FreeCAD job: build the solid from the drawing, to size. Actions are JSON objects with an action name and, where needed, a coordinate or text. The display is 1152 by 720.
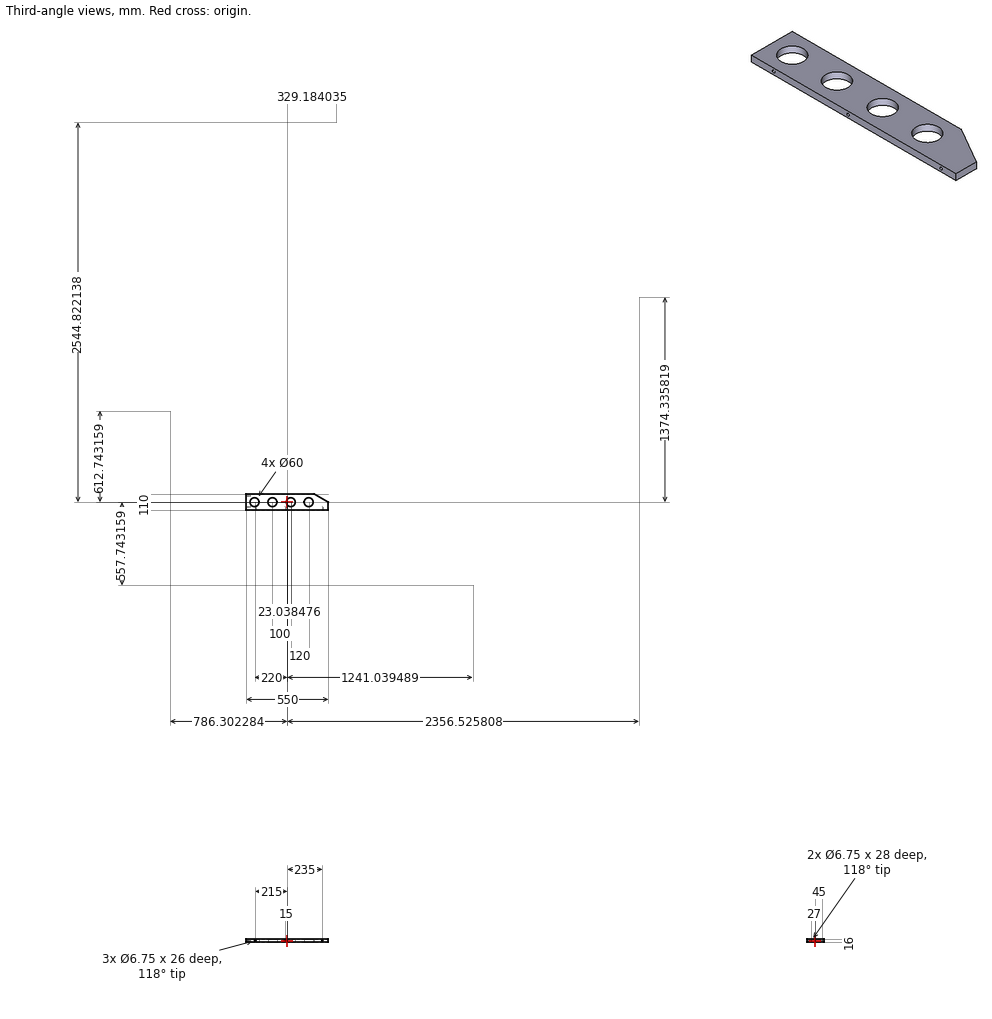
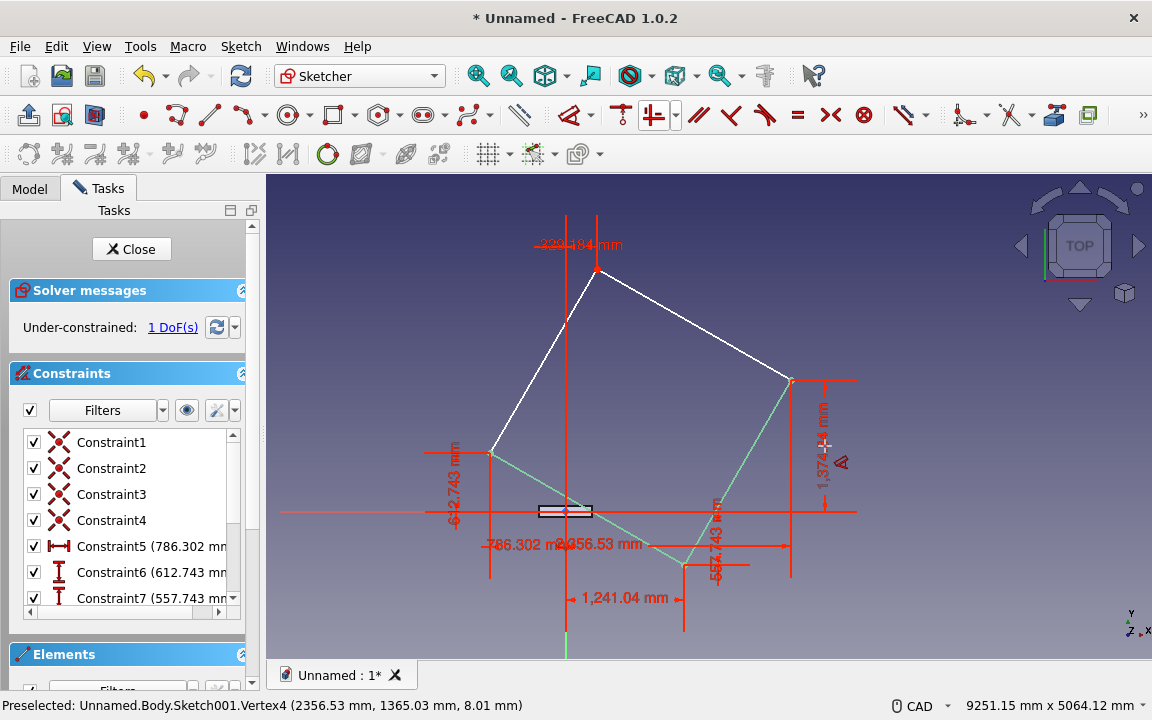
{"action": "left_click", "coordinate": [597, 269]}
{"action": "left_click", "coordinate": [532, 335]}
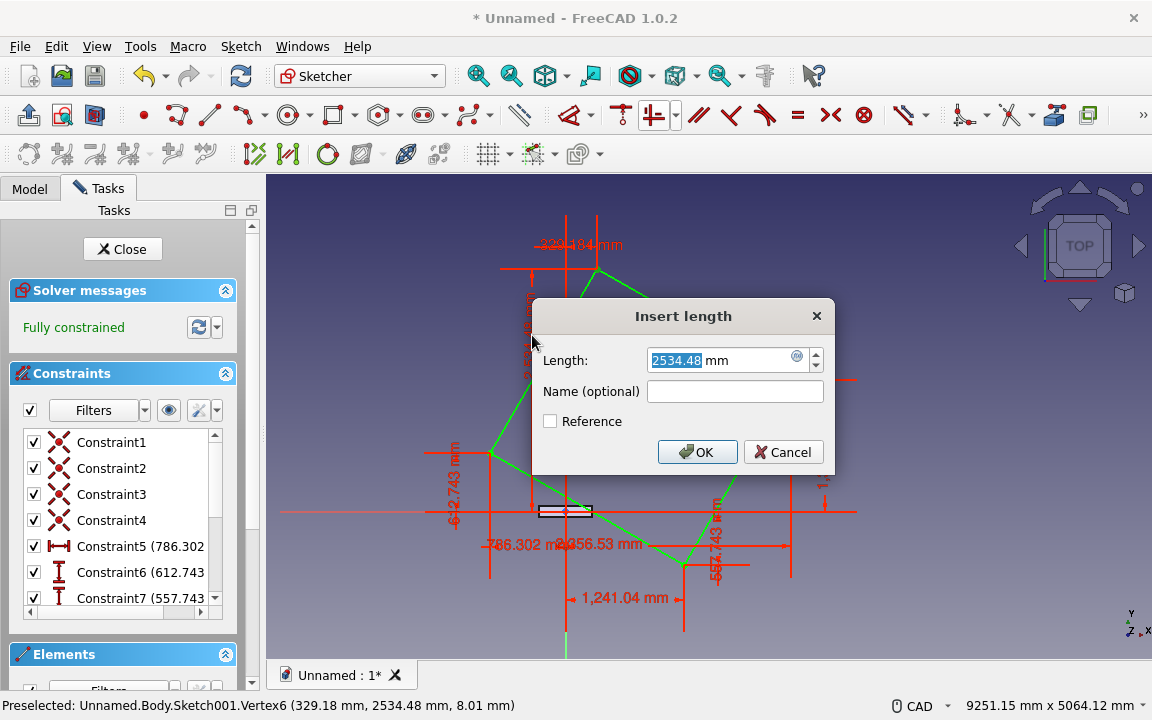
{"action": "type", "text": "2544.822138"}
{"action": "key", "text": "Return"}
{"action": "key", "text": "Escape"}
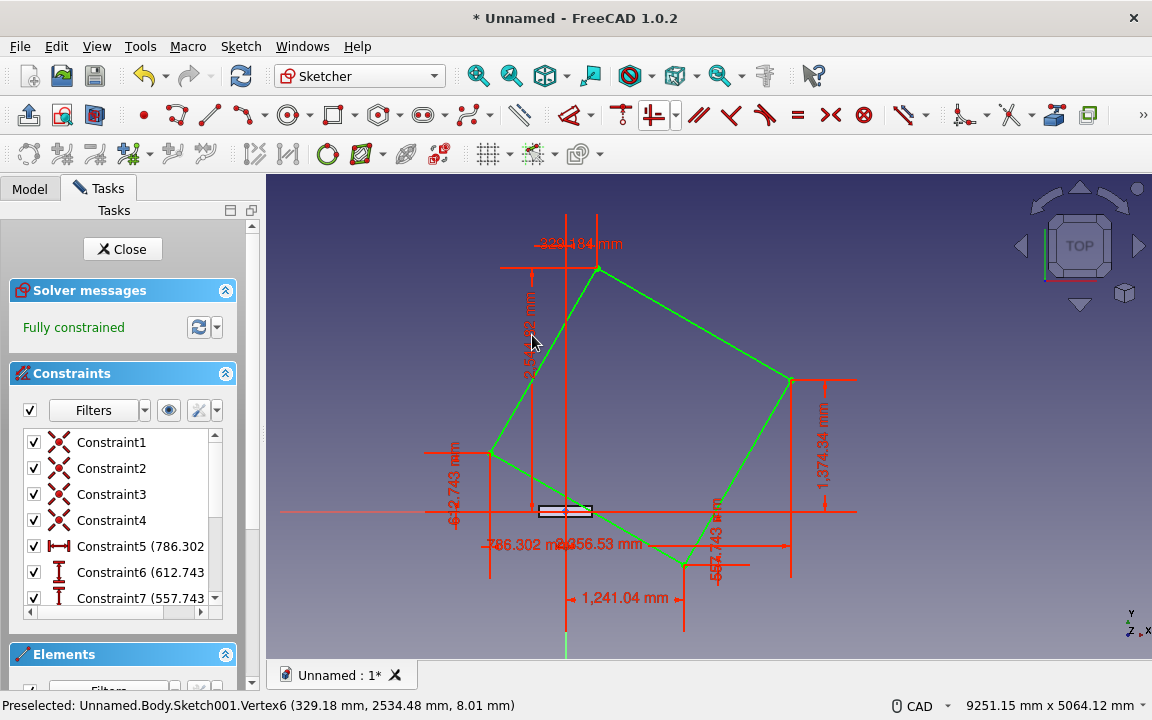
{"action": "left_click", "coordinate": [123, 249]}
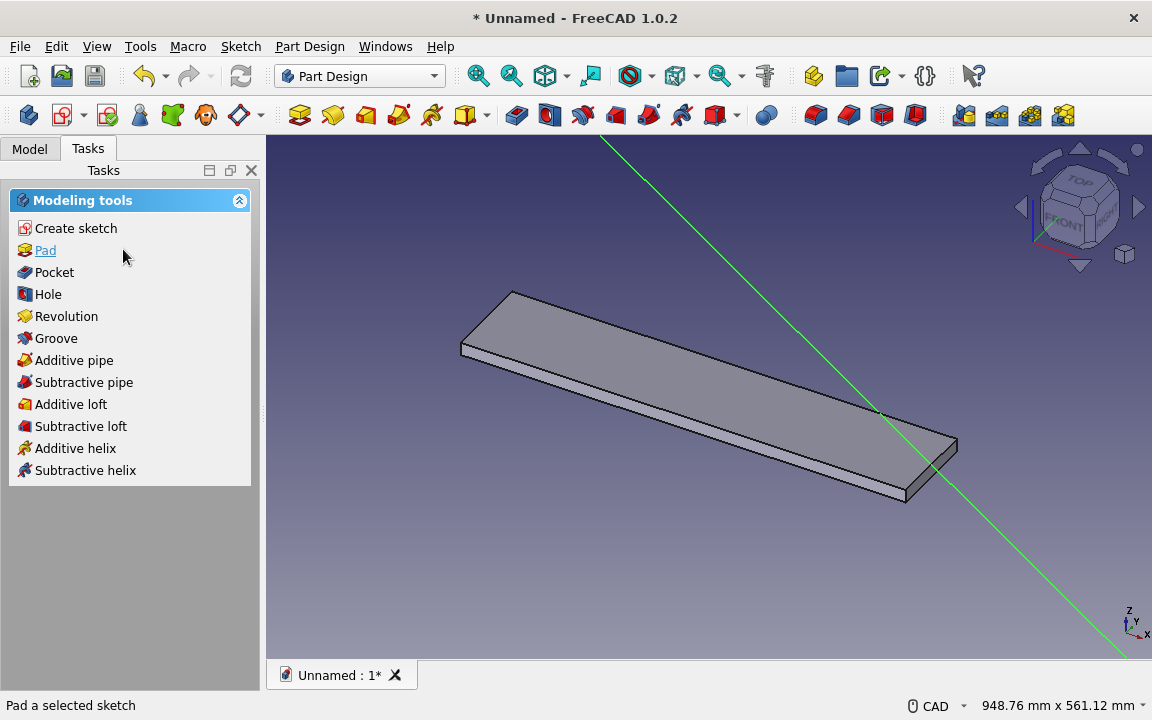
{"action": "left_click", "coordinate": [517, 116]}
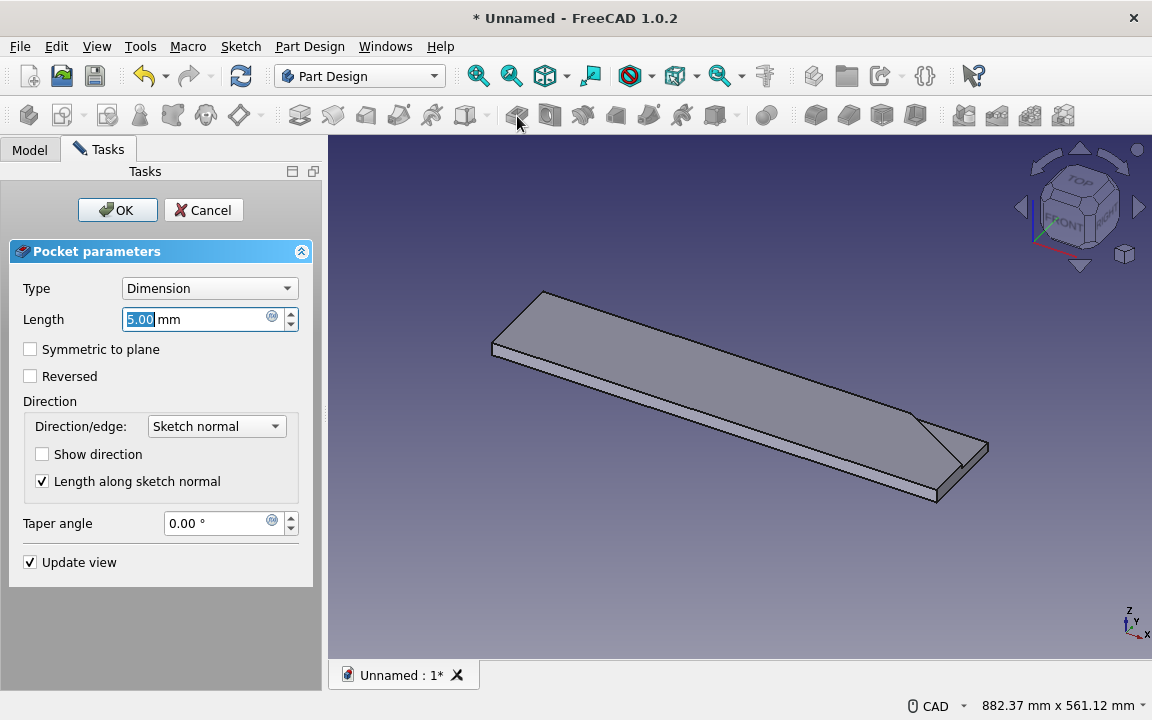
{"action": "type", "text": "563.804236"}
{"action": "key", "text": "Tab"}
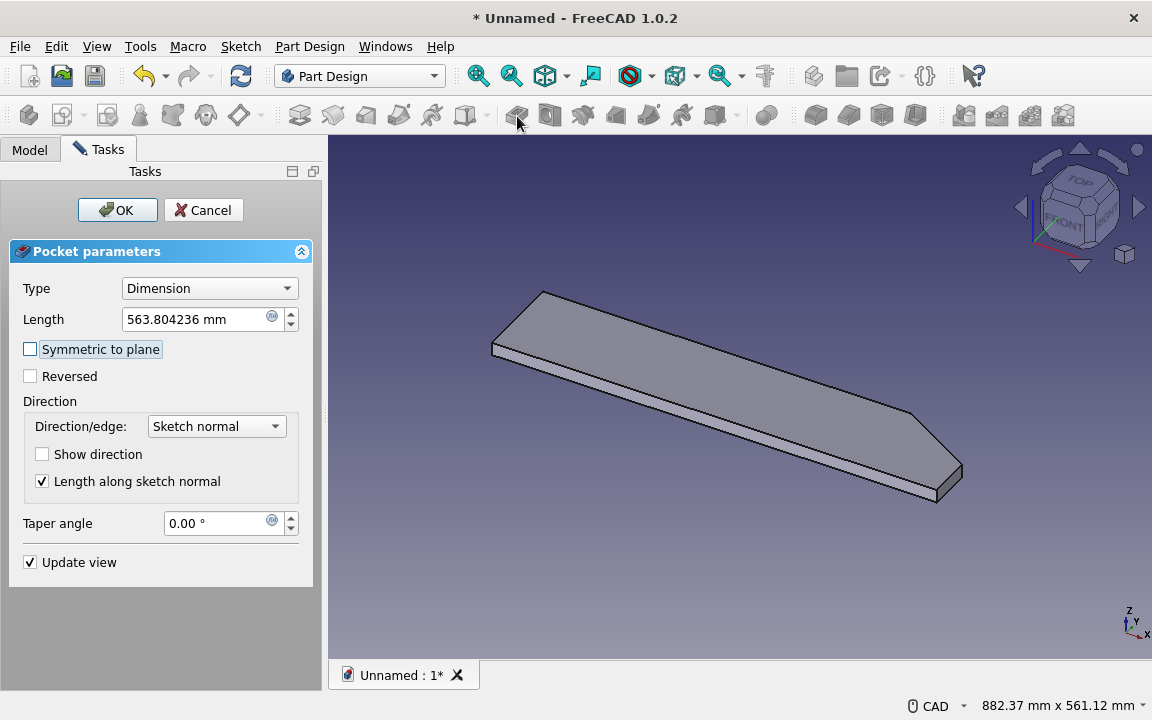
{"action": "left_click", "coordinate": [31, 349]}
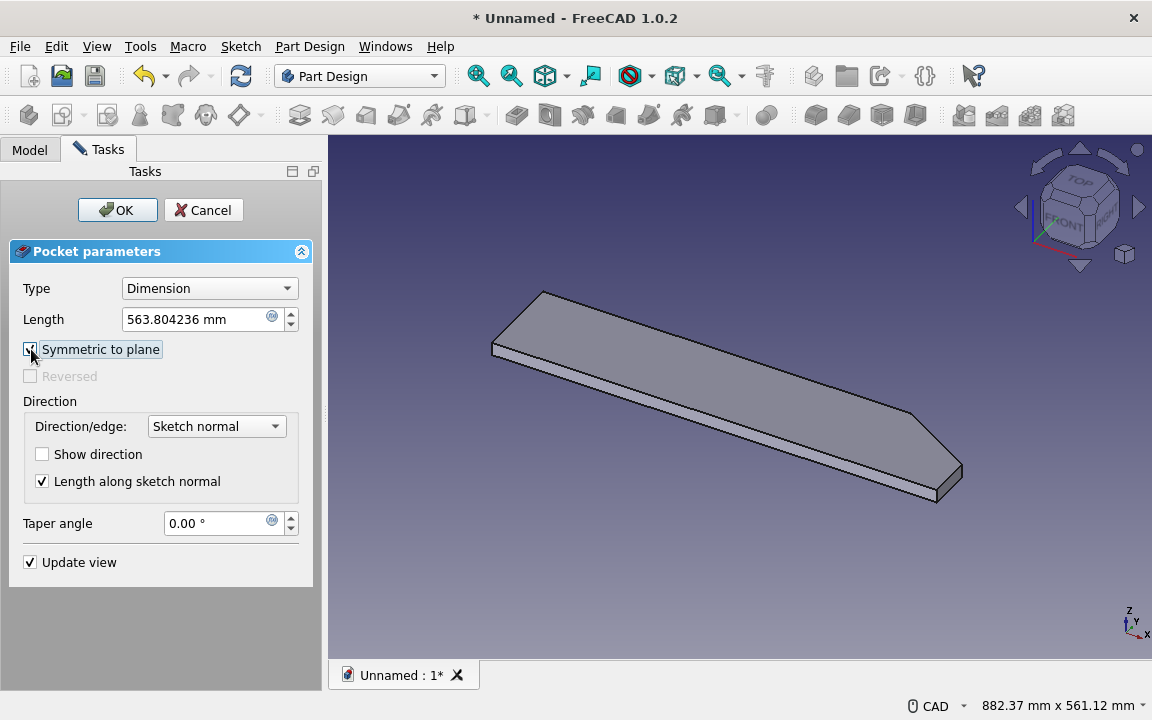
{"action": "left_click", "coordinate": [118, 210]}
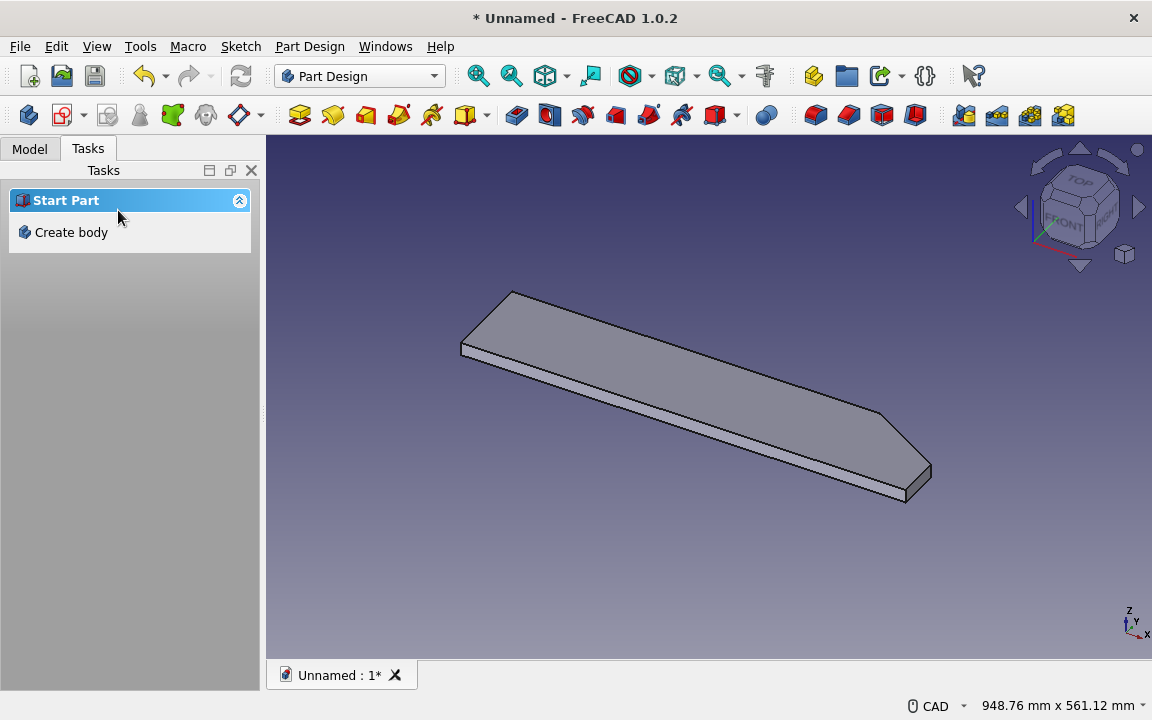
{"action": "key", "text": "0"}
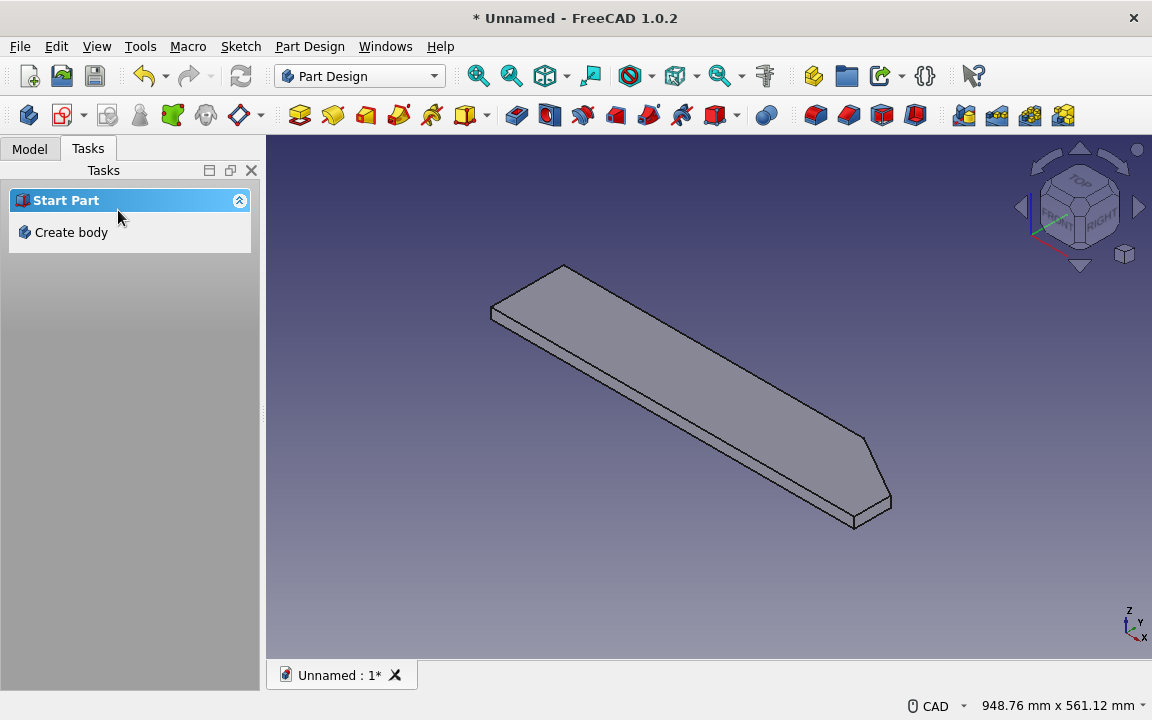
{"action": "key", "text": "1"}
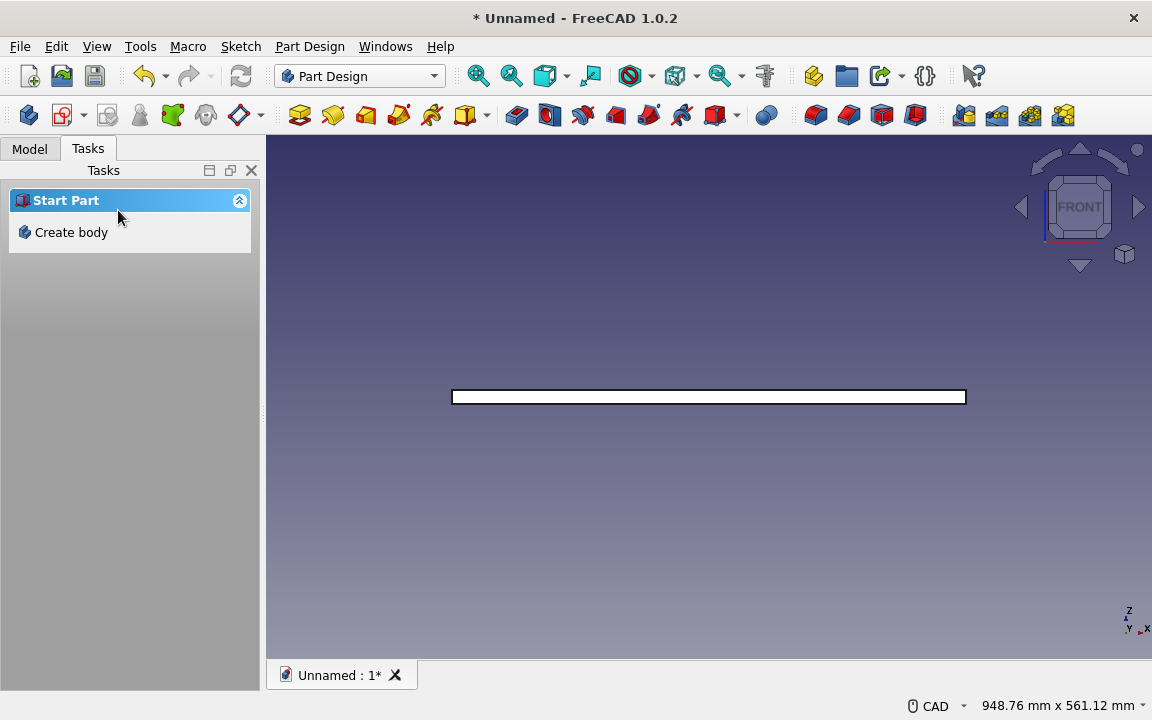
{"action": "key", "text": "2"}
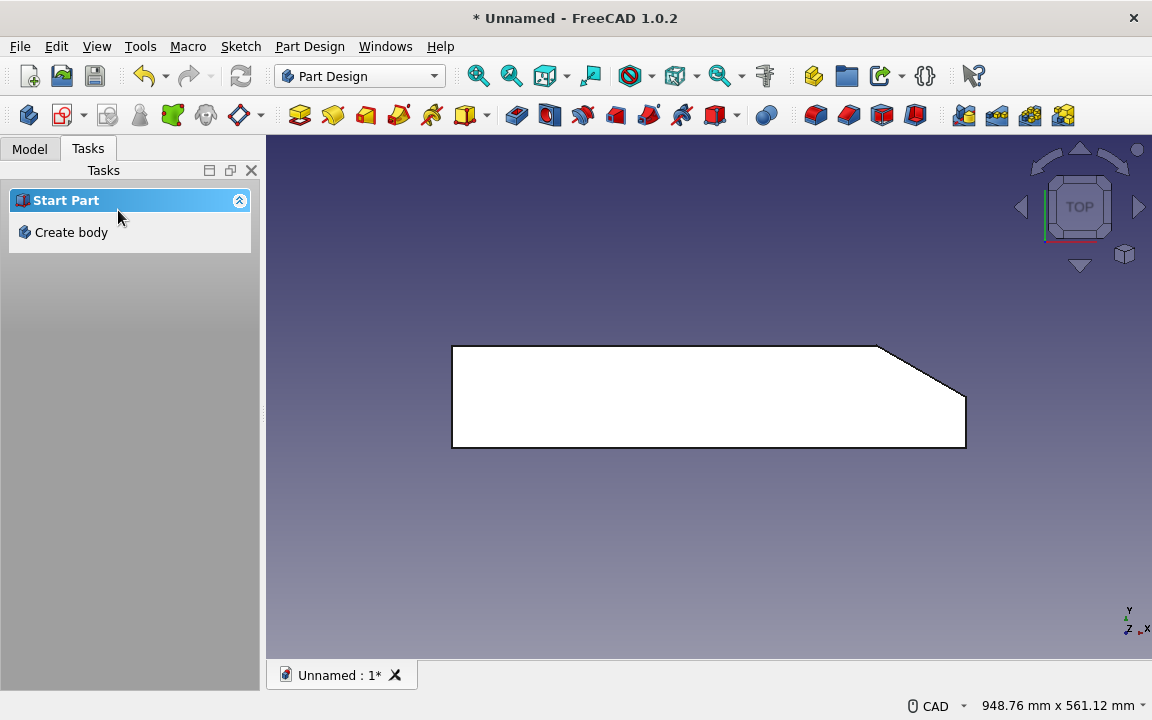
{"action": "left_click", "coordinate": [30, 148]}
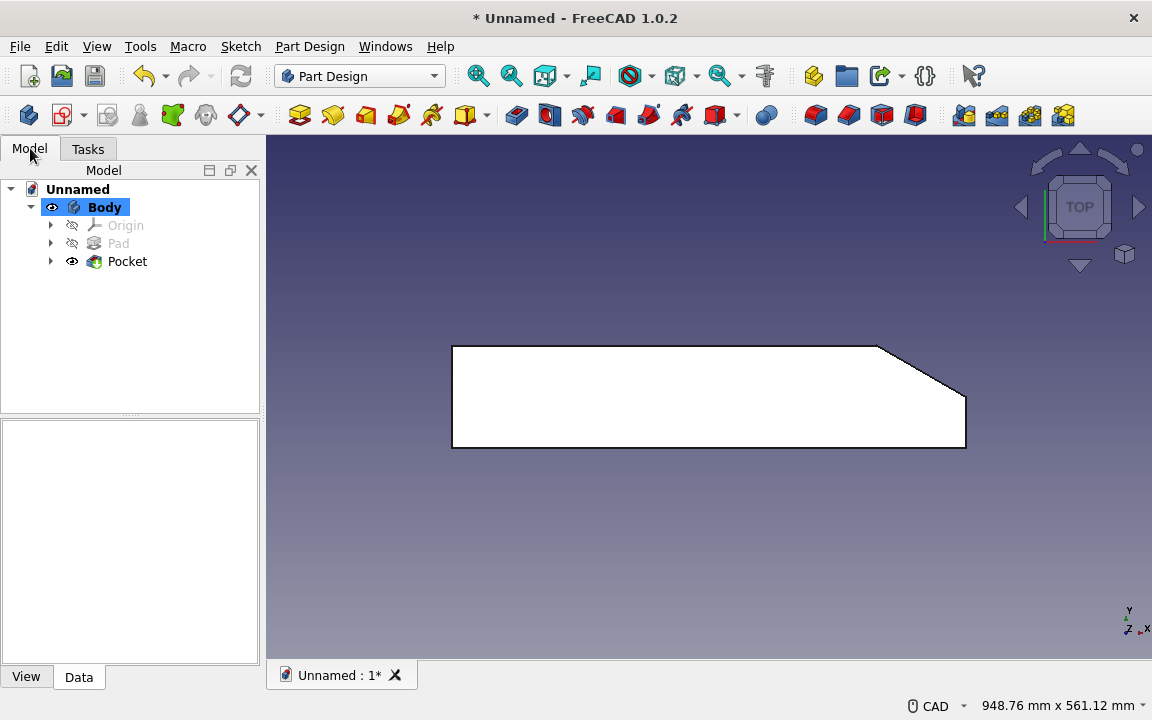
{"action": "left_click", "coordinate": [51, 225]}